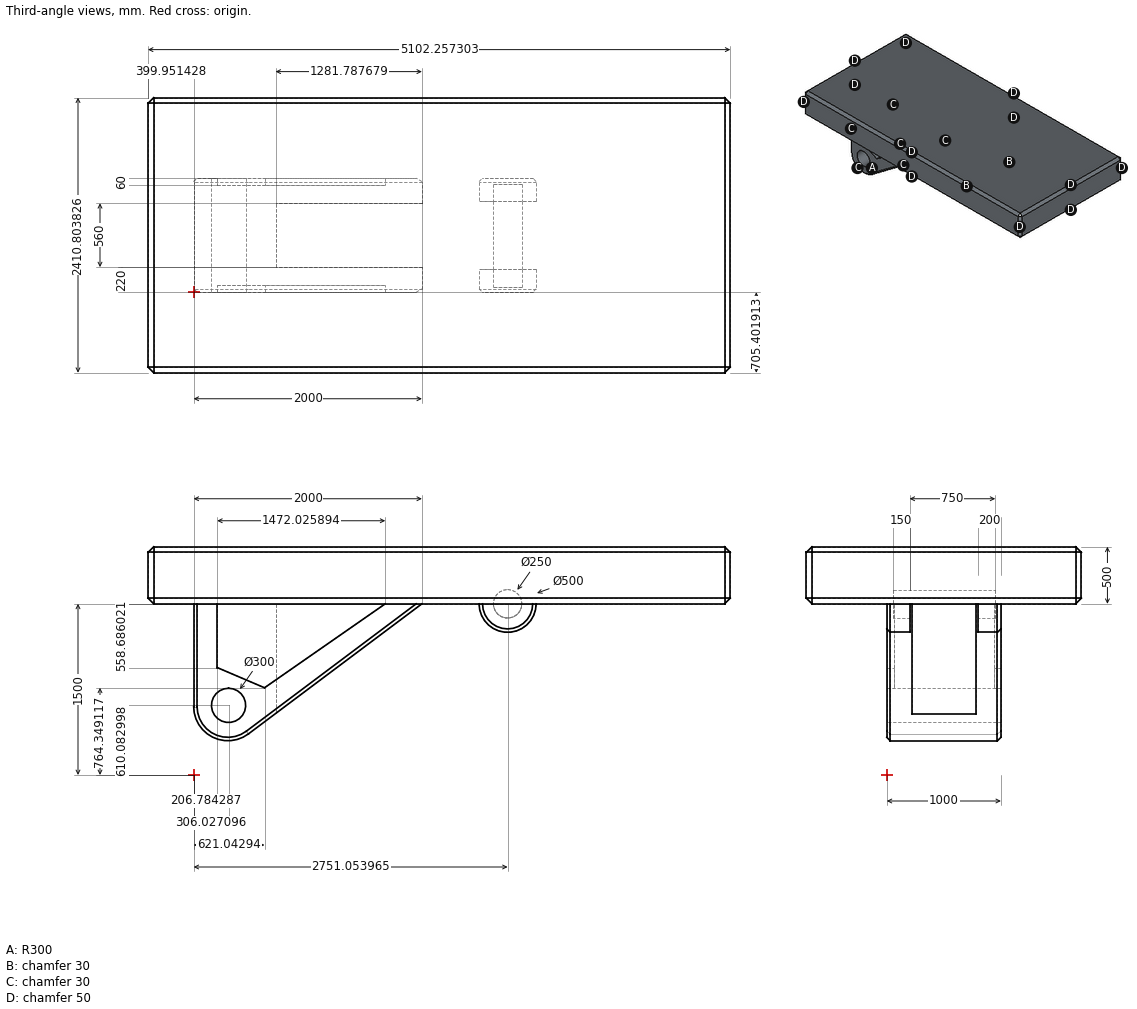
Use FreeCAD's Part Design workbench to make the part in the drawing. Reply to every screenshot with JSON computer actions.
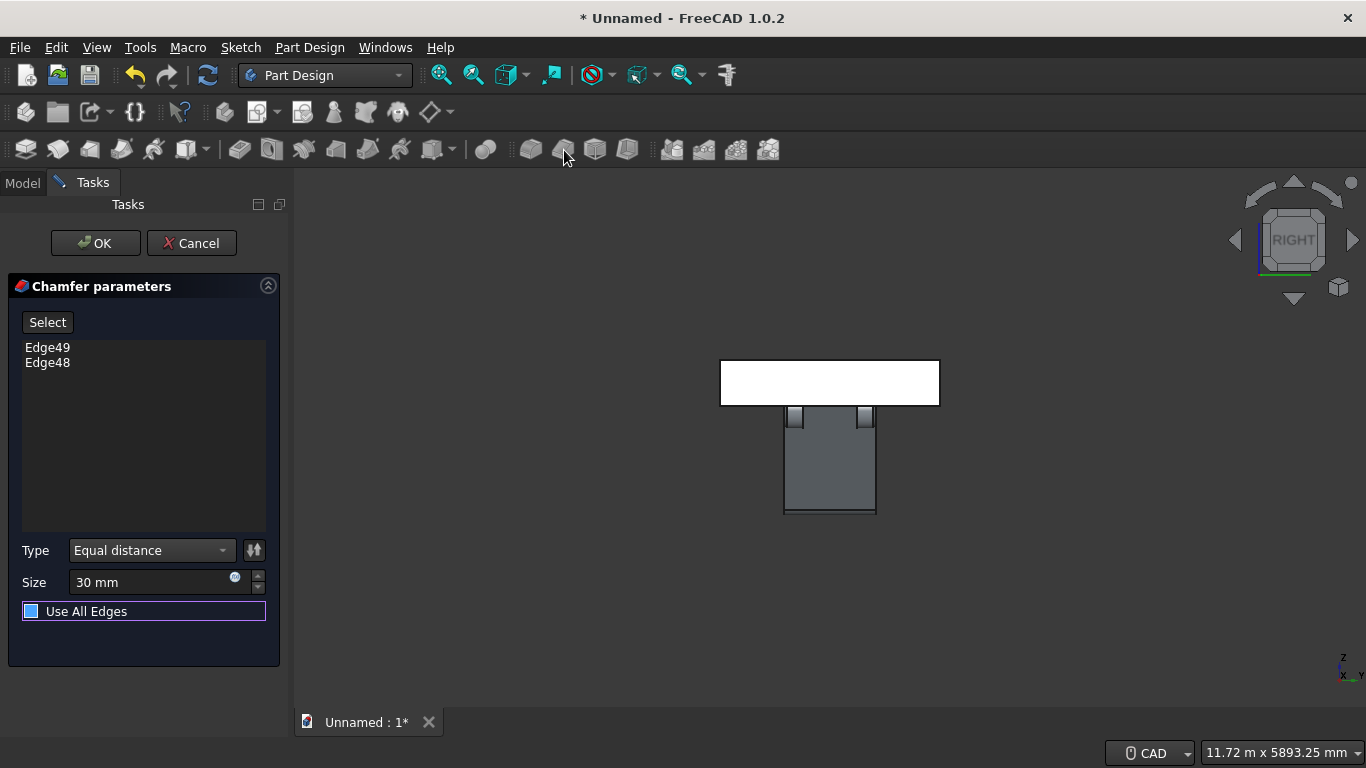
{"action": "left_click", "coordinate": [96, 243]}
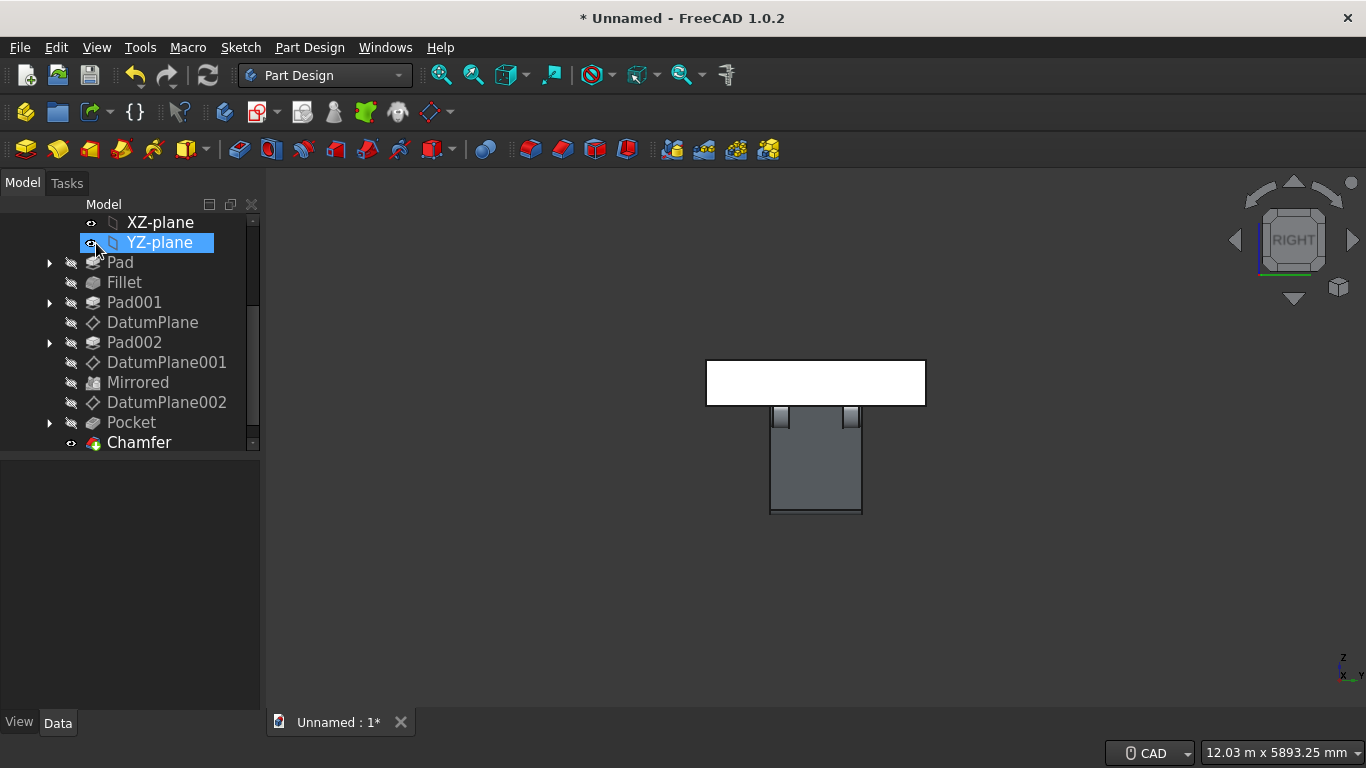
{"action": "left_click", "coordinate": [442, 76]}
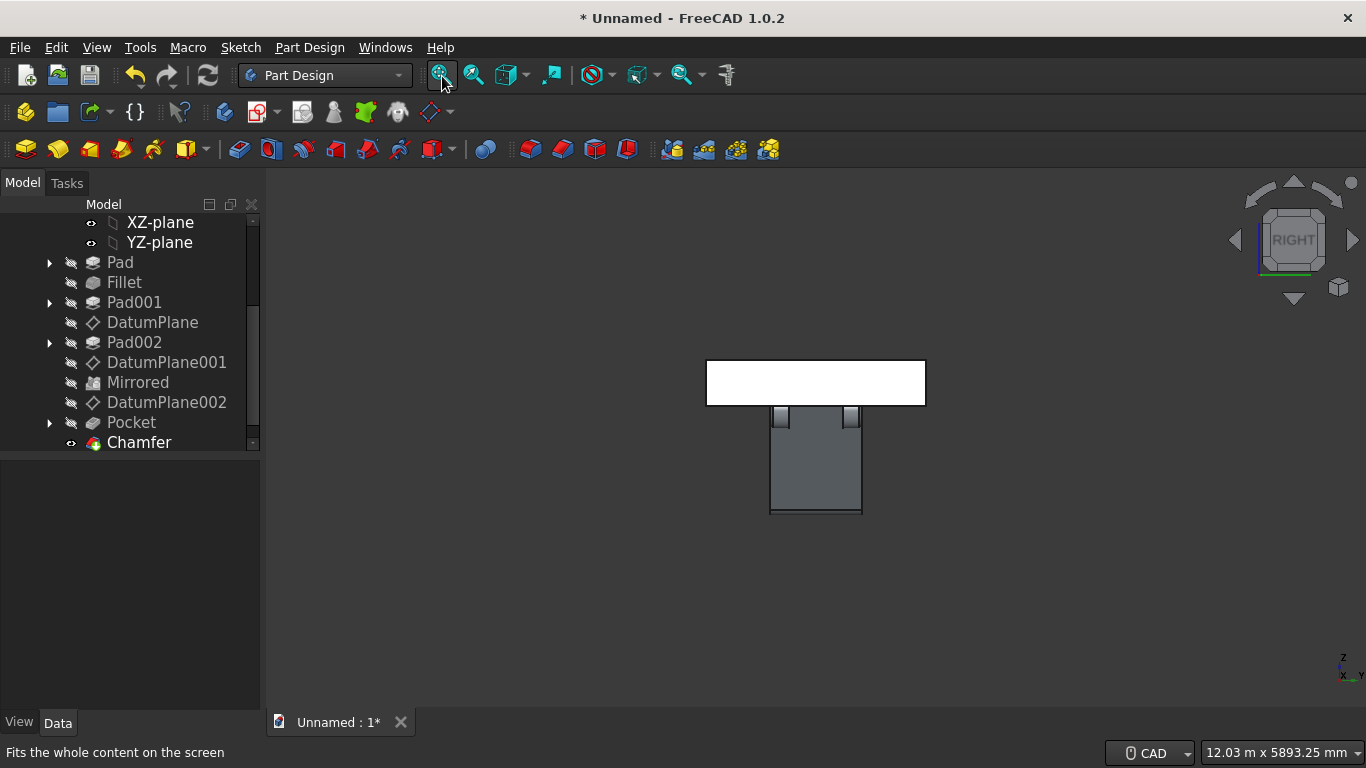
{"action": "left_click", "coordinate": [770, 457]}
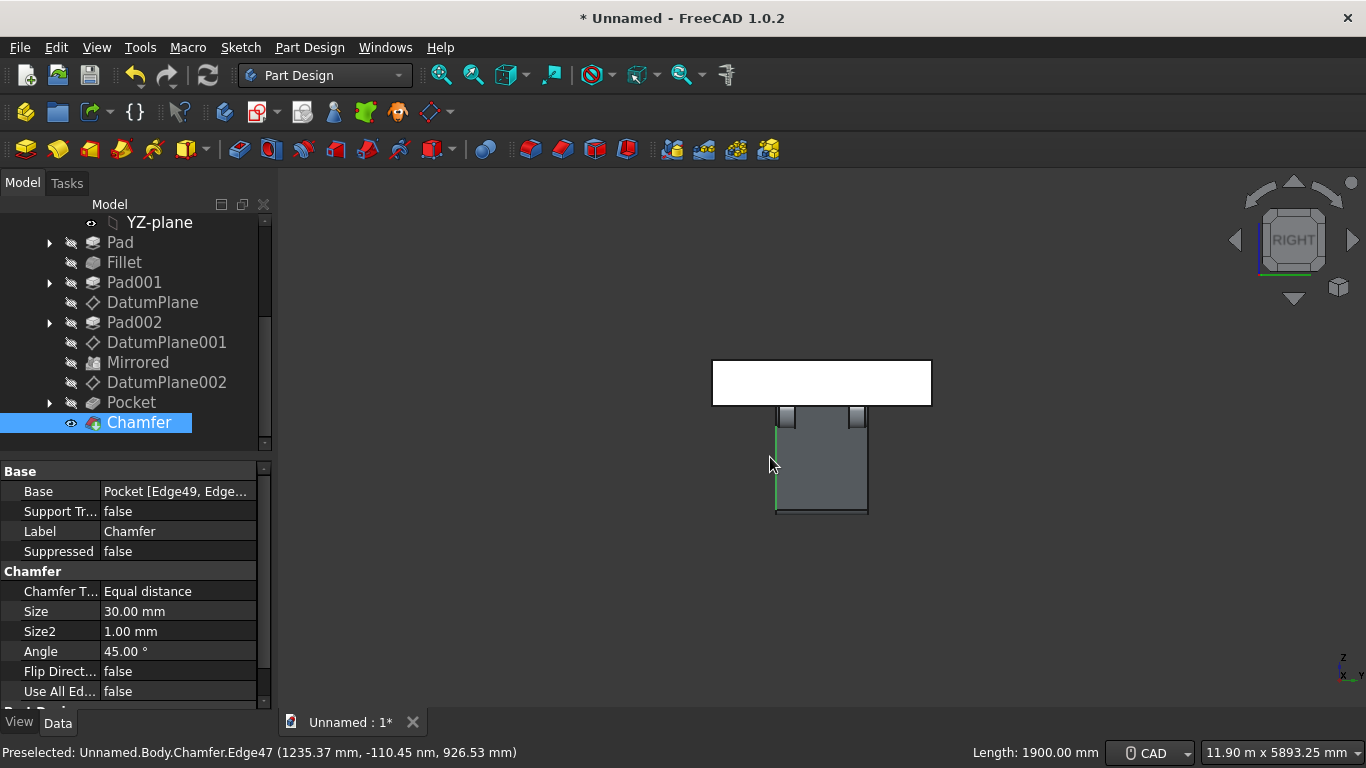
{"action": "left_click", "coordinate": [868, 457], "text": "ctrl"}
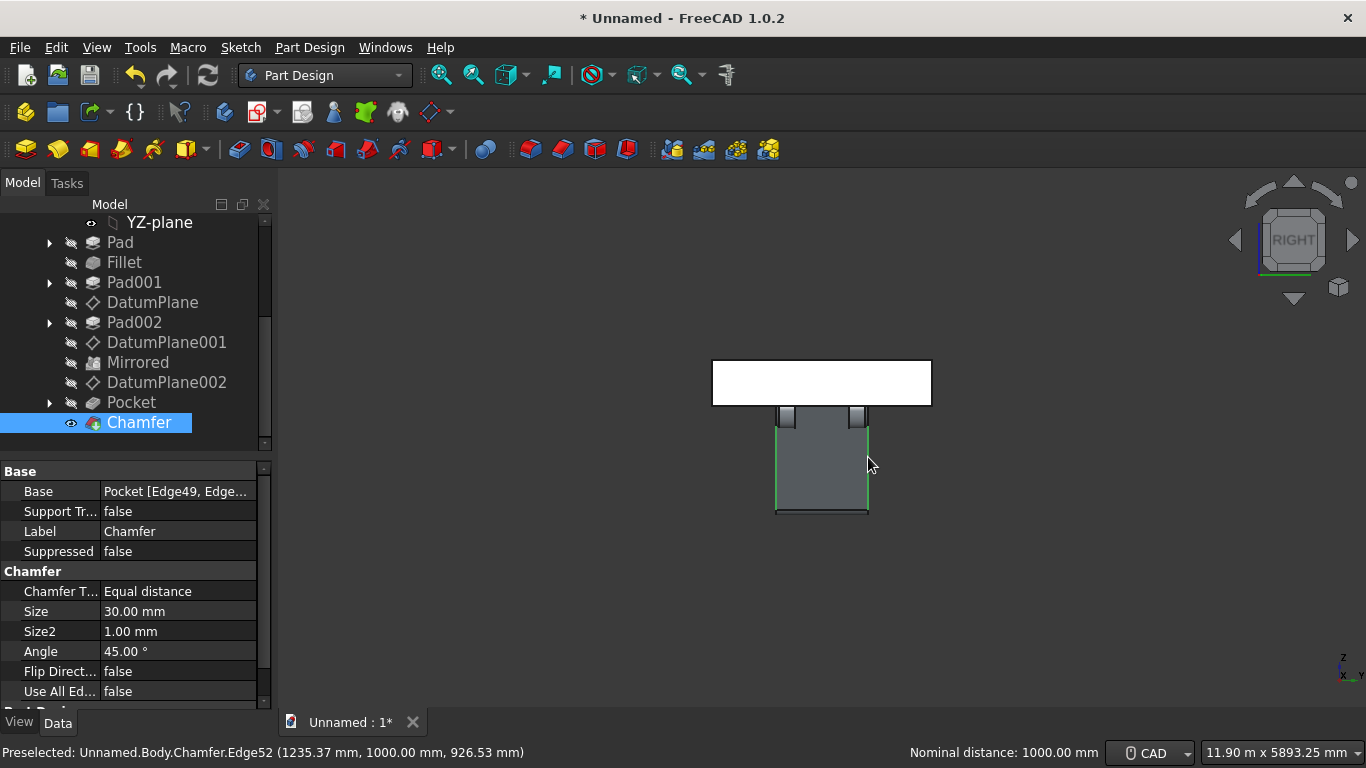
{"action": "key", "text": "0"}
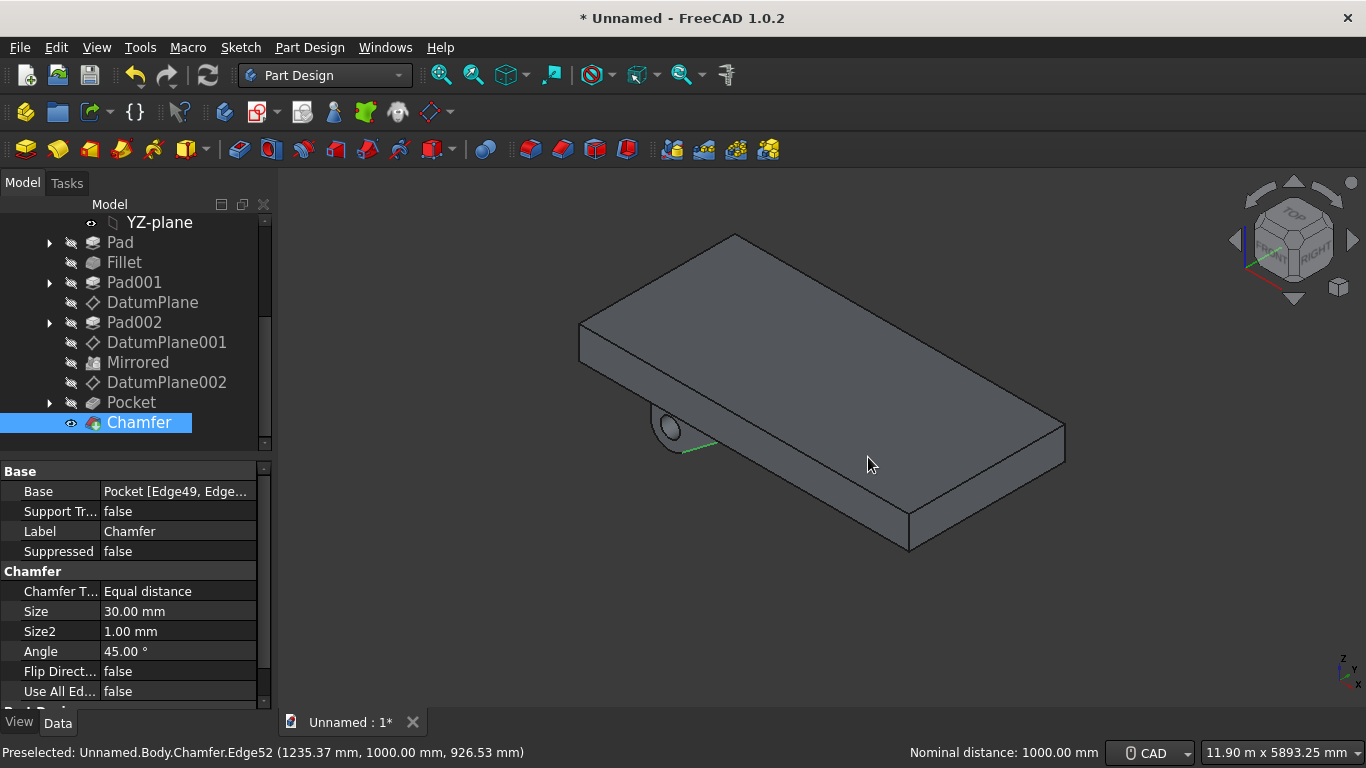
{"action": "left_click", "coordinate": [665, 446], "text": "ctrl"}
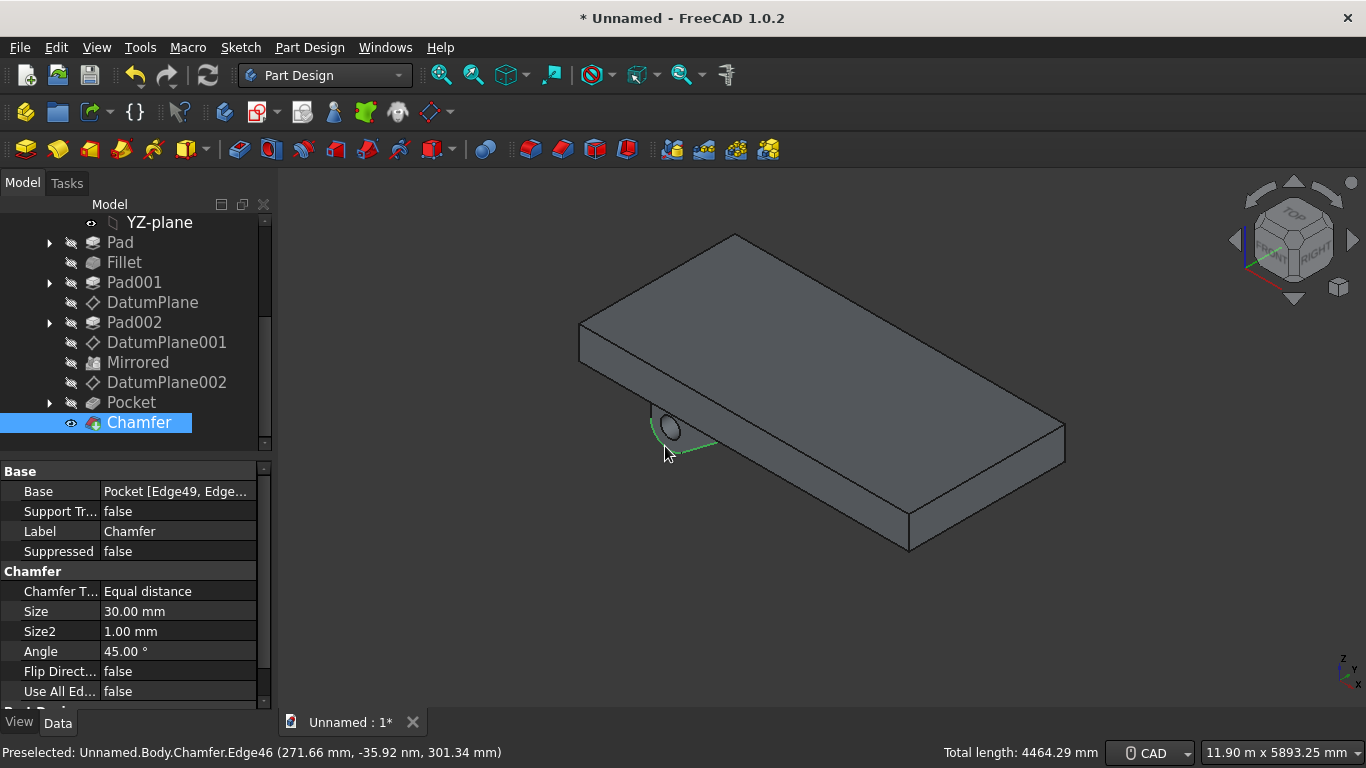
{"action": "key", "text": "2"}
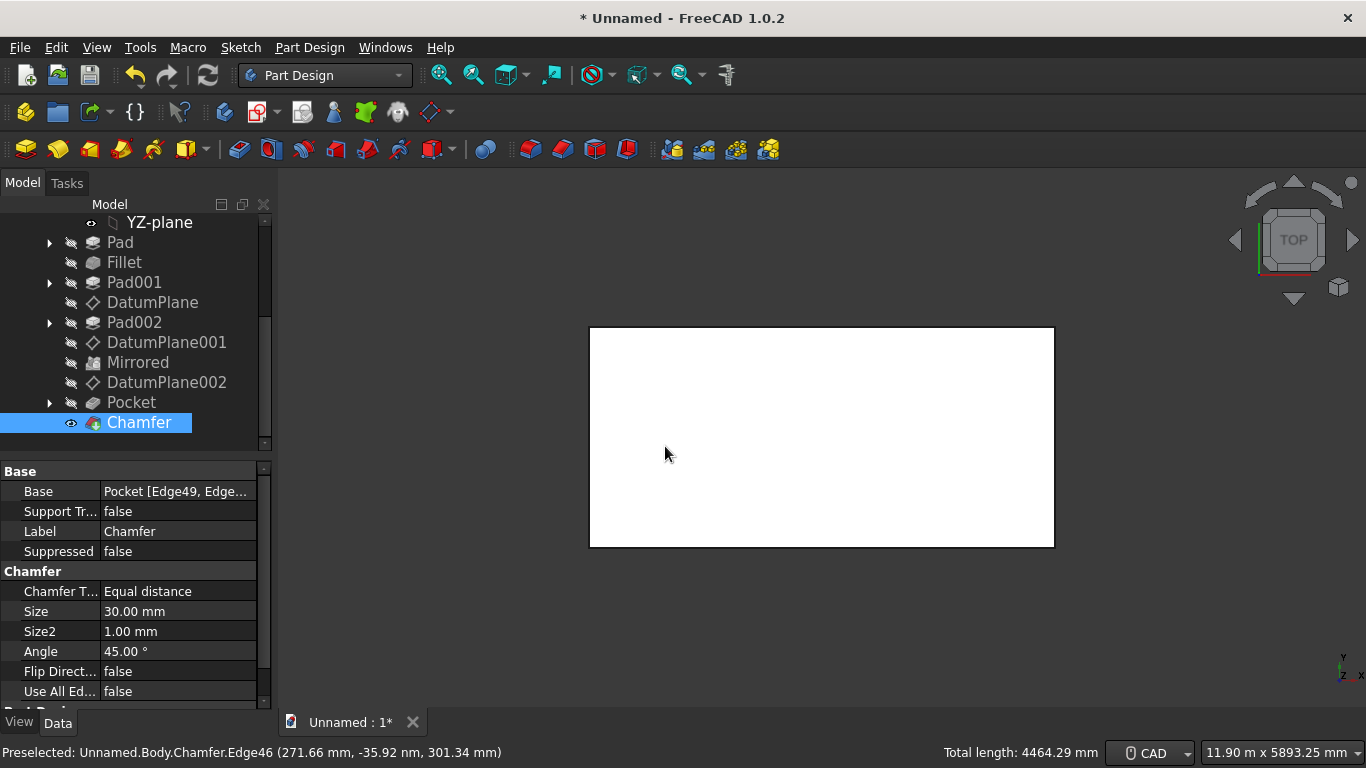
{"action": "left_click", "coordinate": [442, 76]}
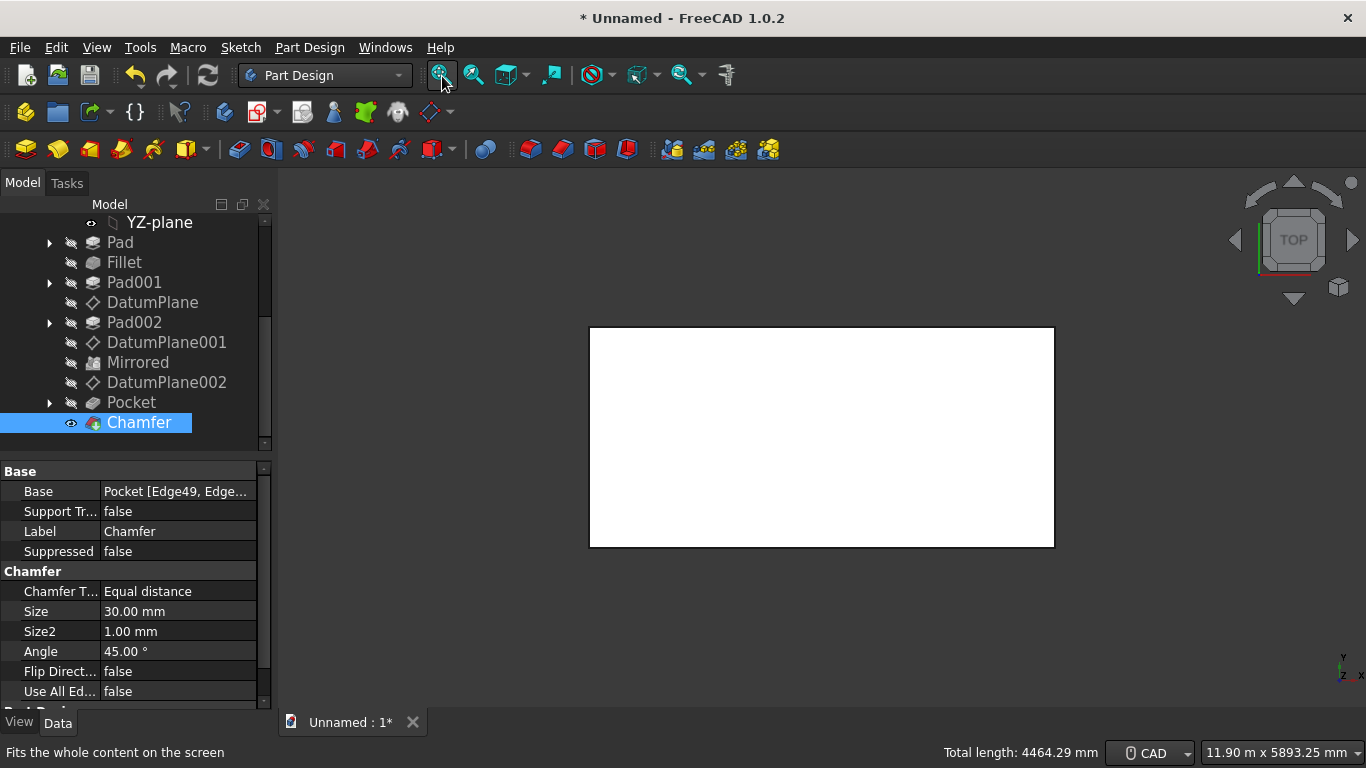
{"action": "key", "text": "1"}